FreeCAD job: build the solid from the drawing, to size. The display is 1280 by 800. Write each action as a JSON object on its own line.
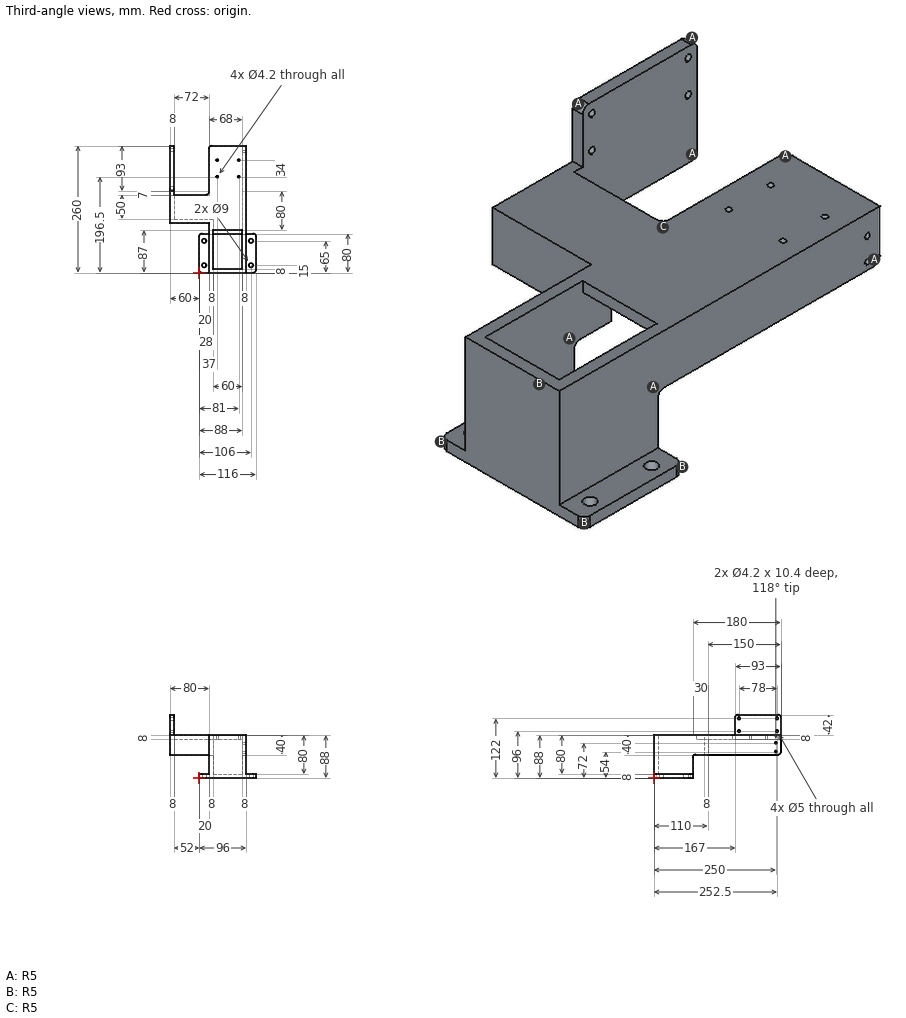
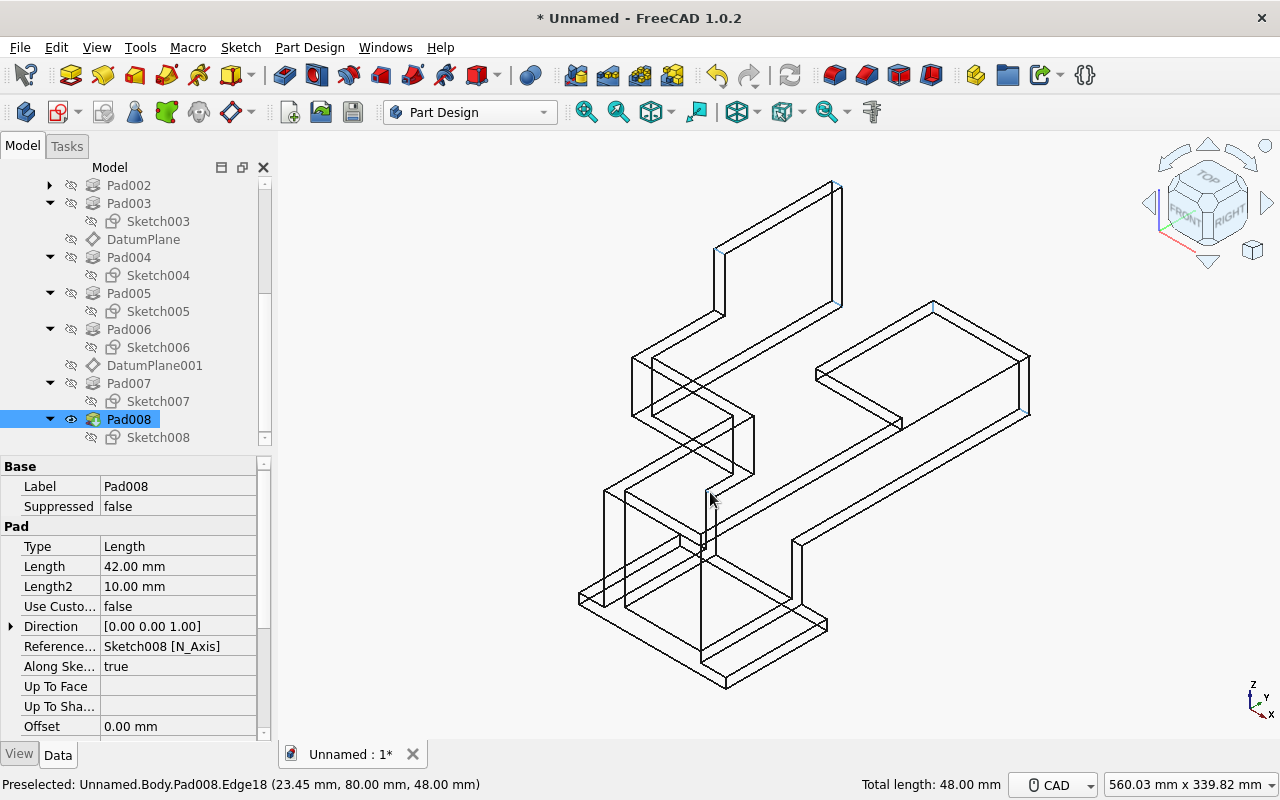
{"action": "left_click", "coordinate": [796, 542], "text": "ctrl"}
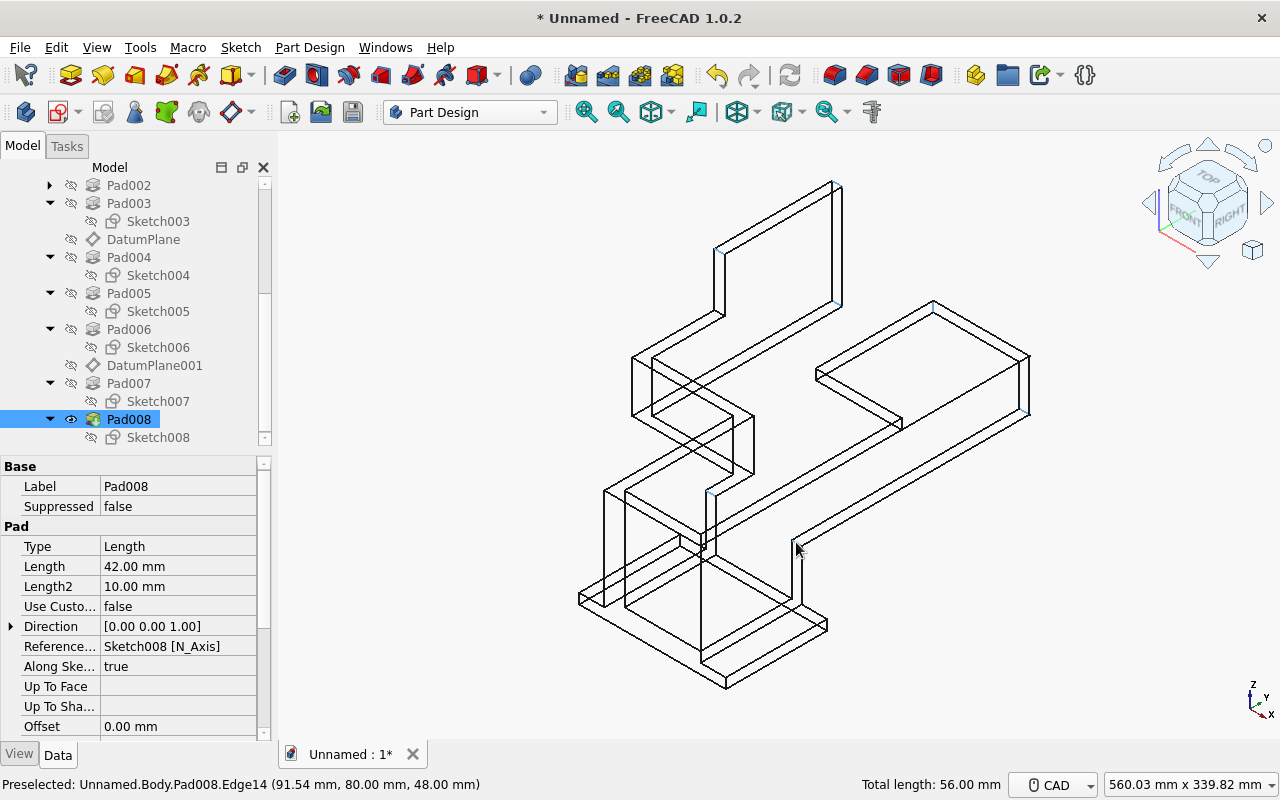
{"action": "key", "text": "v 1"}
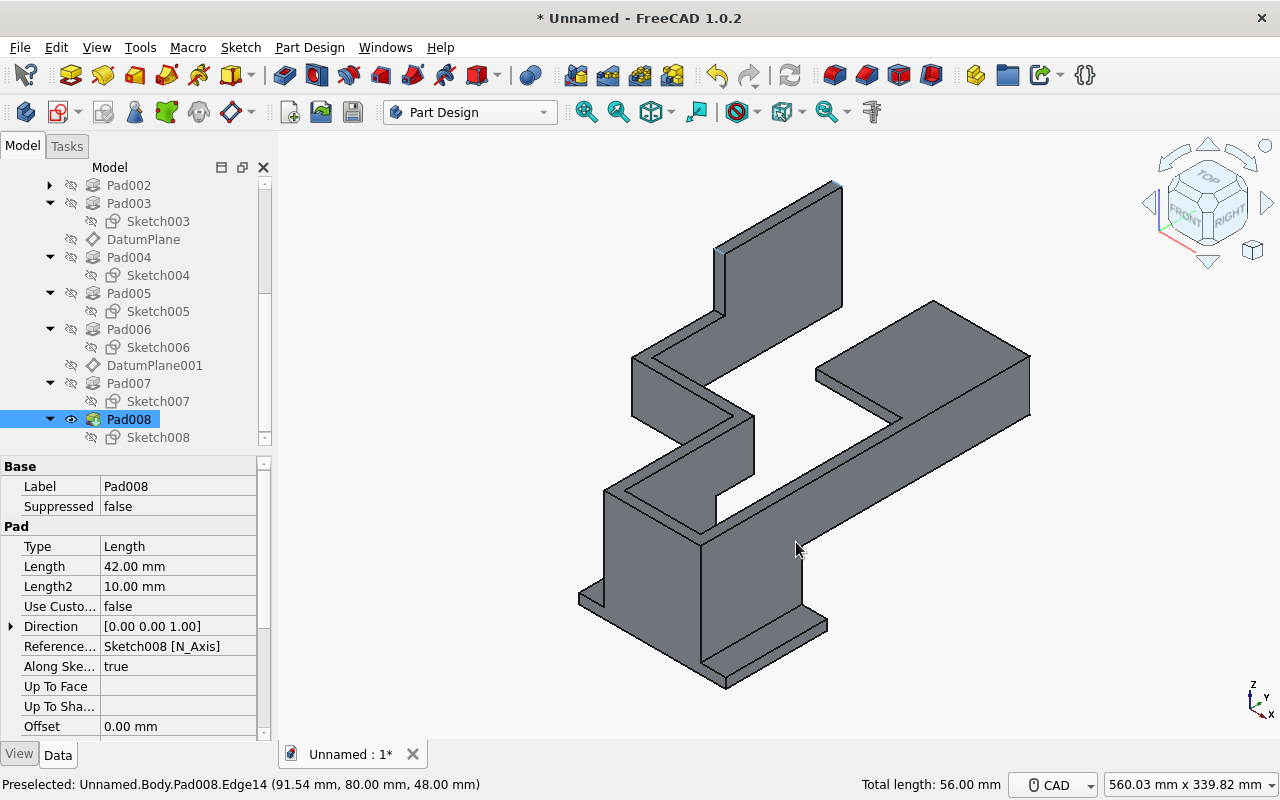
{"action": "left_click", "coordinate": [836, 76]}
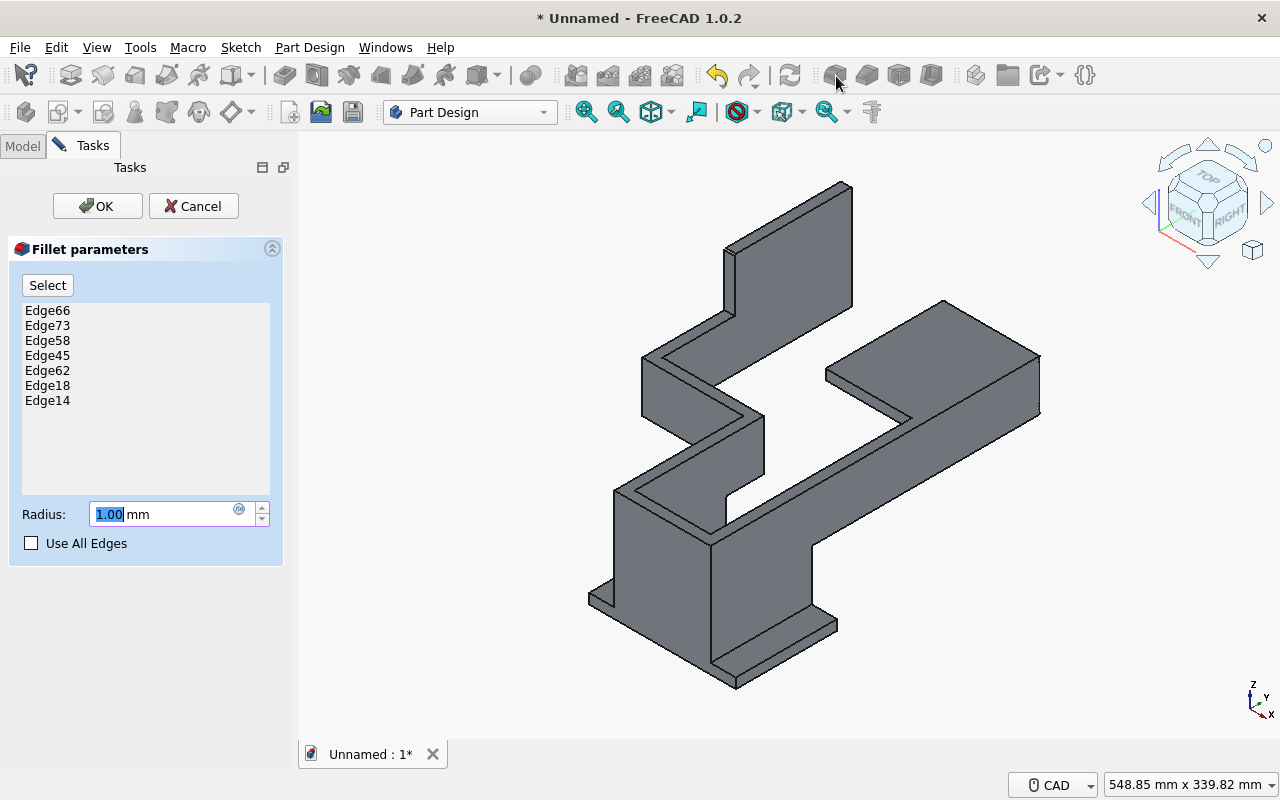
{"action": "type", "text": "5"}
{"action": "key", "text": "Tab"}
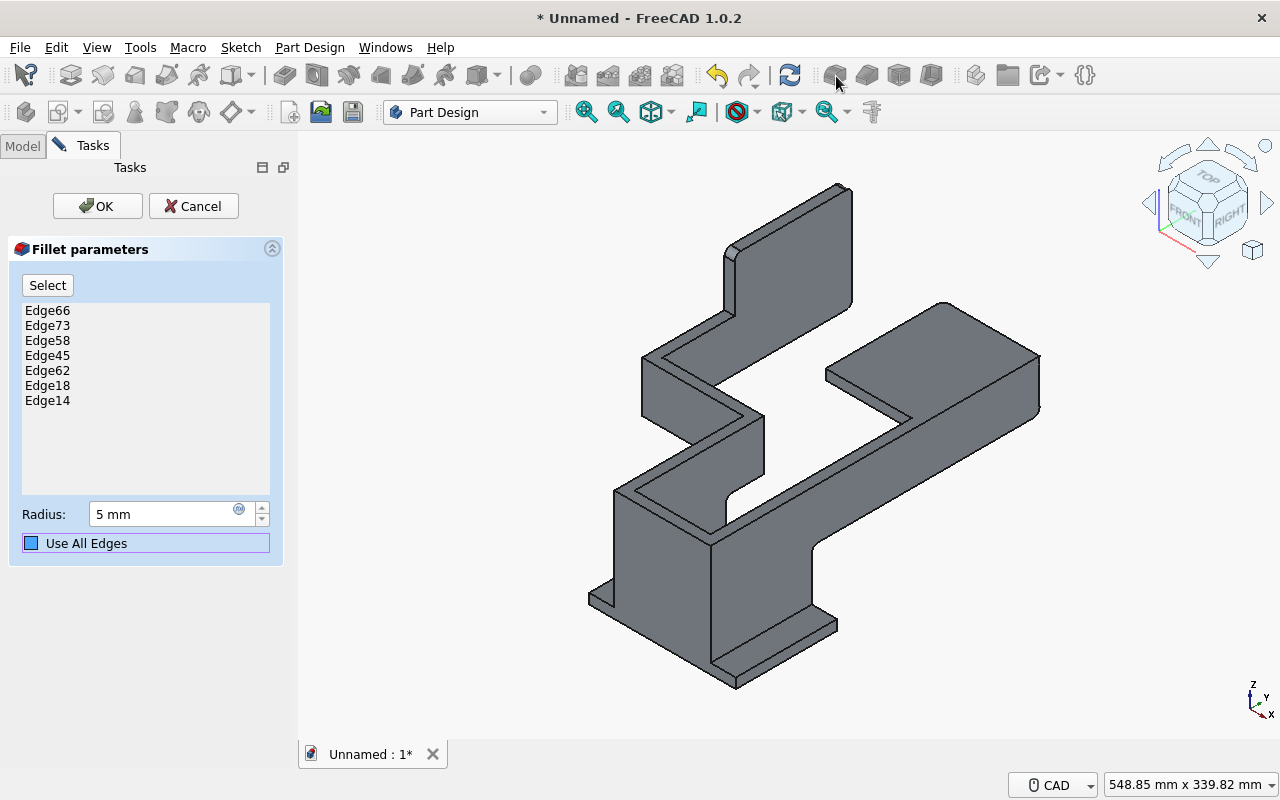
{"action": "left_click", "coordinate": [98, 206]}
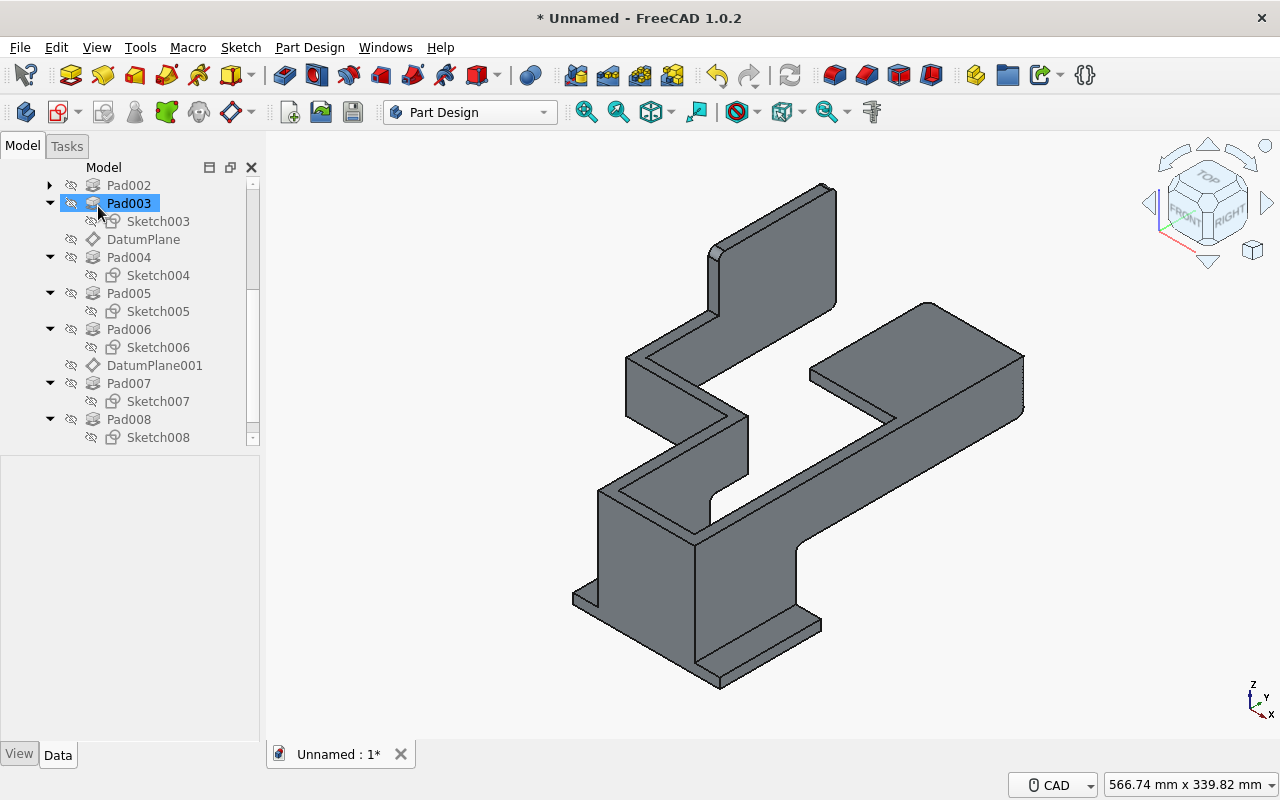
{"action": "left_click", "coordinate": [720, 684]}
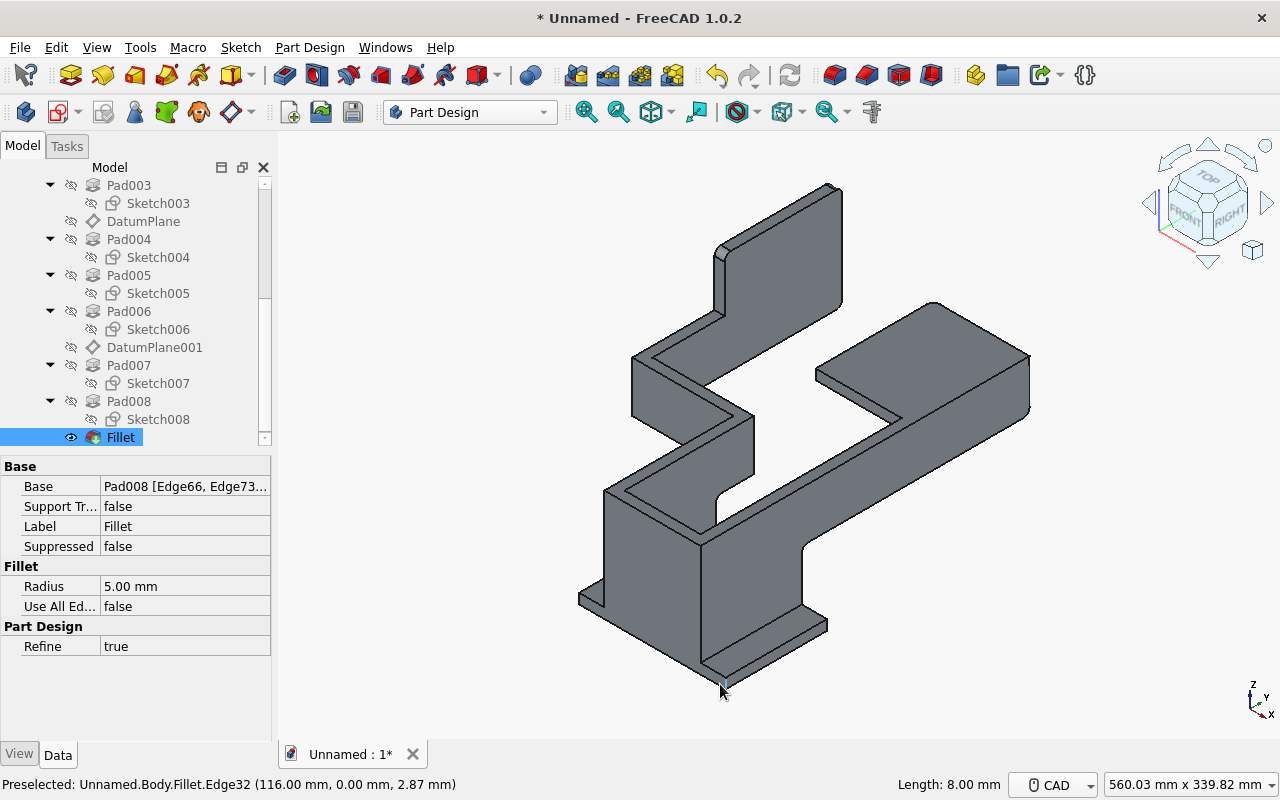
{"action": "scroll", "coordinate": [680, 539], "scroll_direction": "up", "scroll_amount": 6}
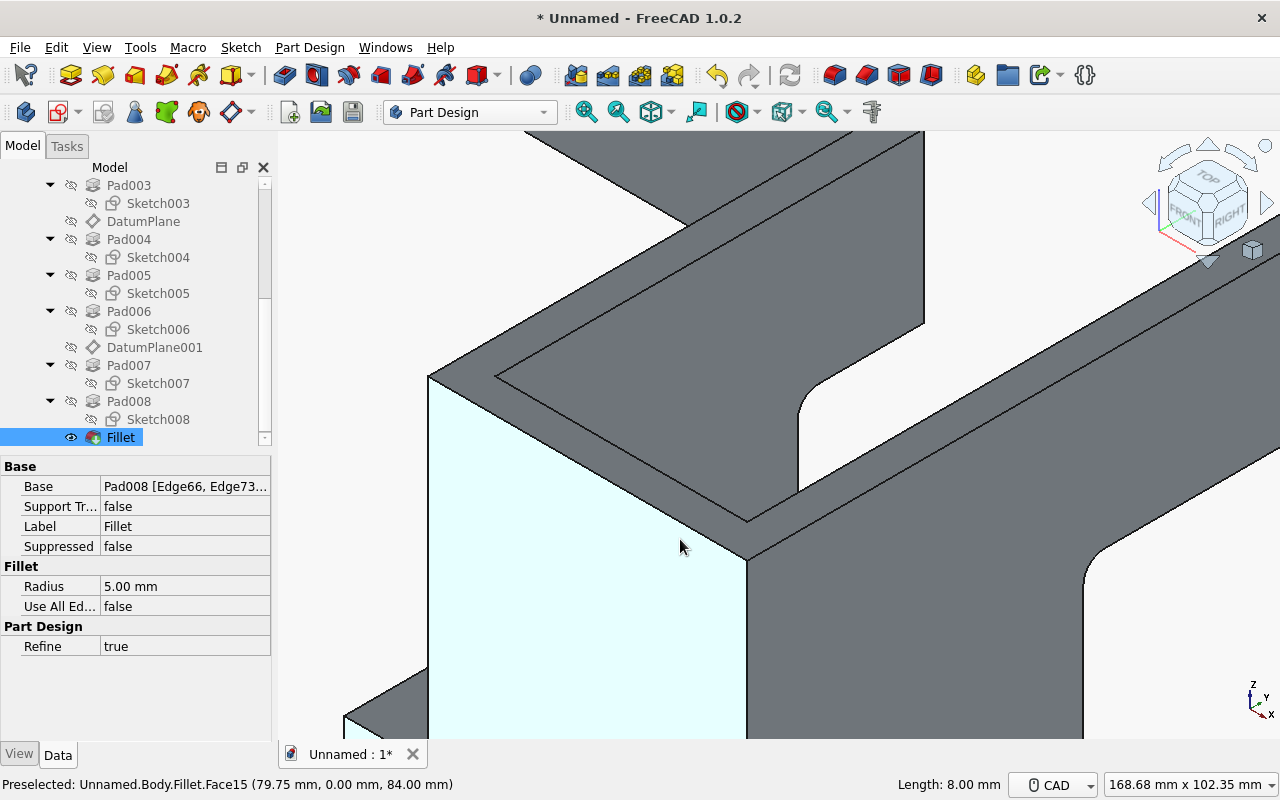
{"action": "left_click", "coordinate": [588, 112]}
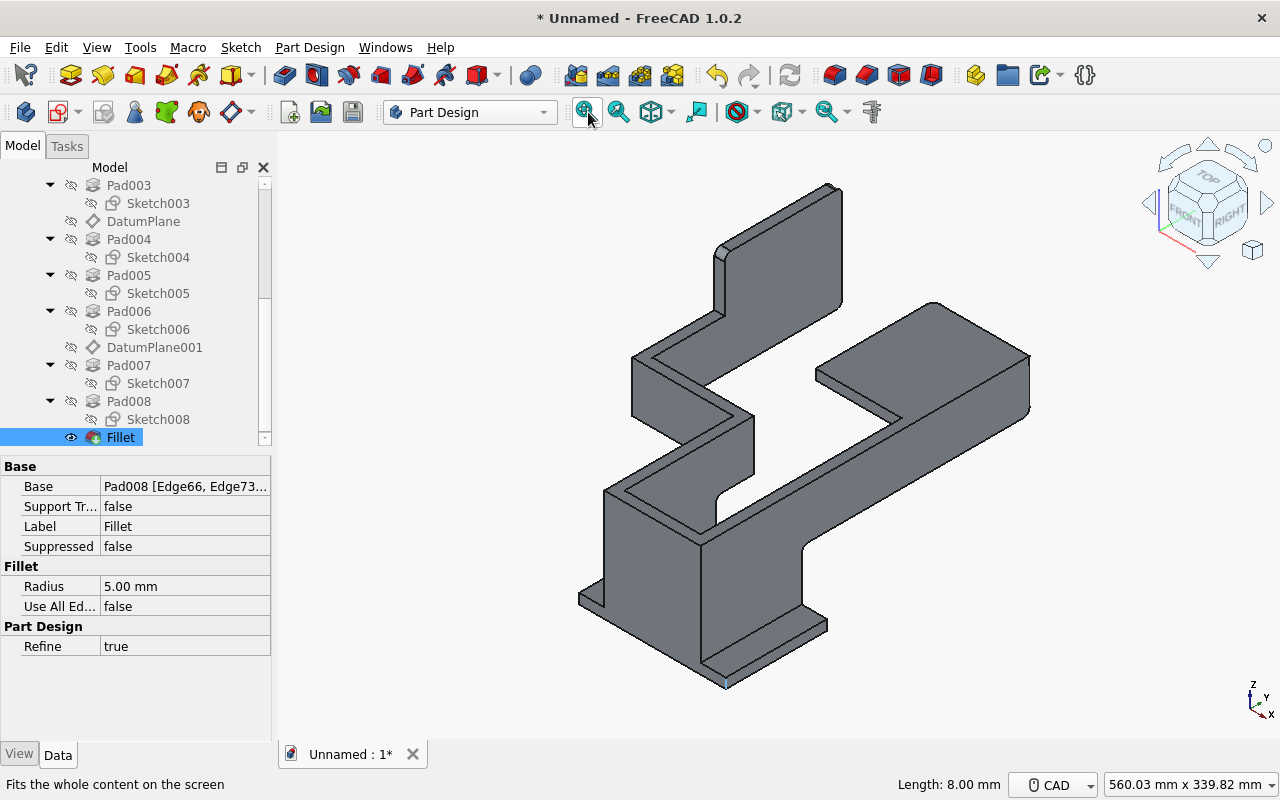
{"action": "key", "text": "2"}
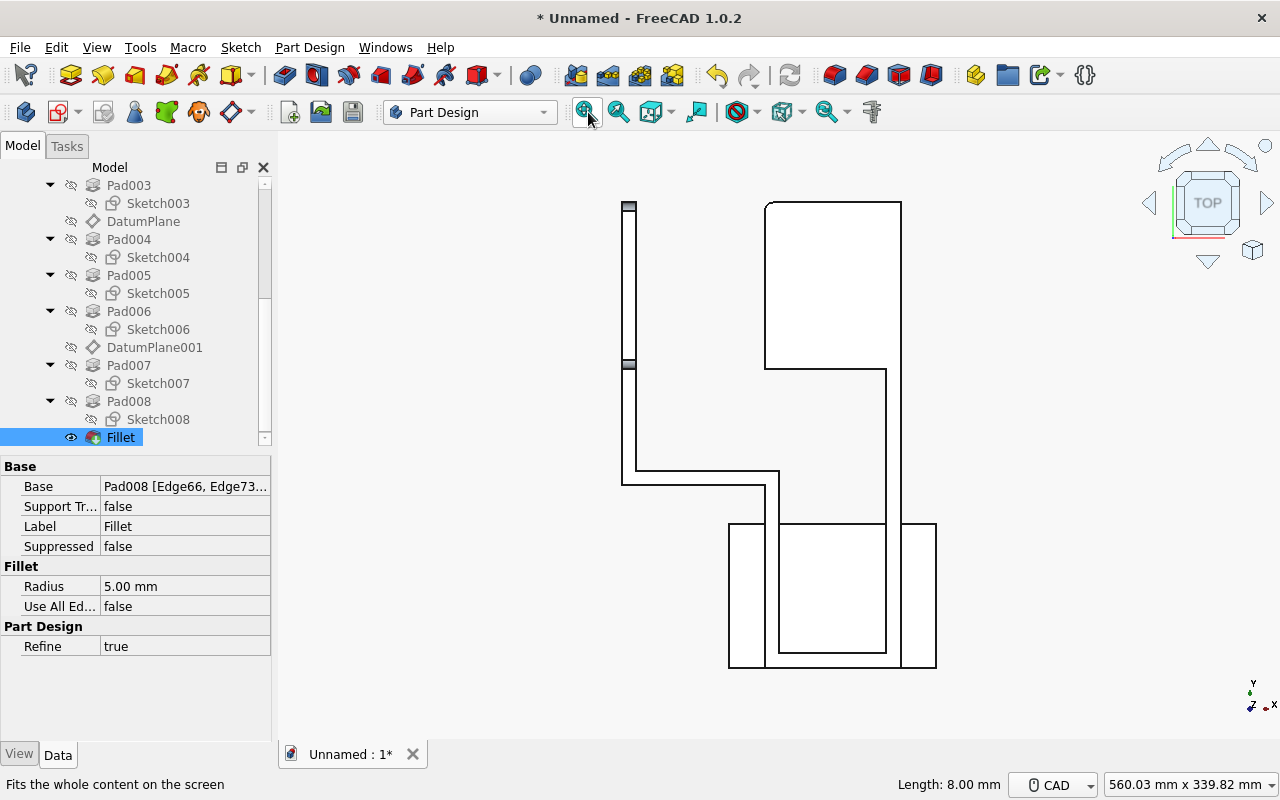
{"action": "scroll", "coordinate": [729, 523], "scroll_direction": "up", "scroll_amount": 6}